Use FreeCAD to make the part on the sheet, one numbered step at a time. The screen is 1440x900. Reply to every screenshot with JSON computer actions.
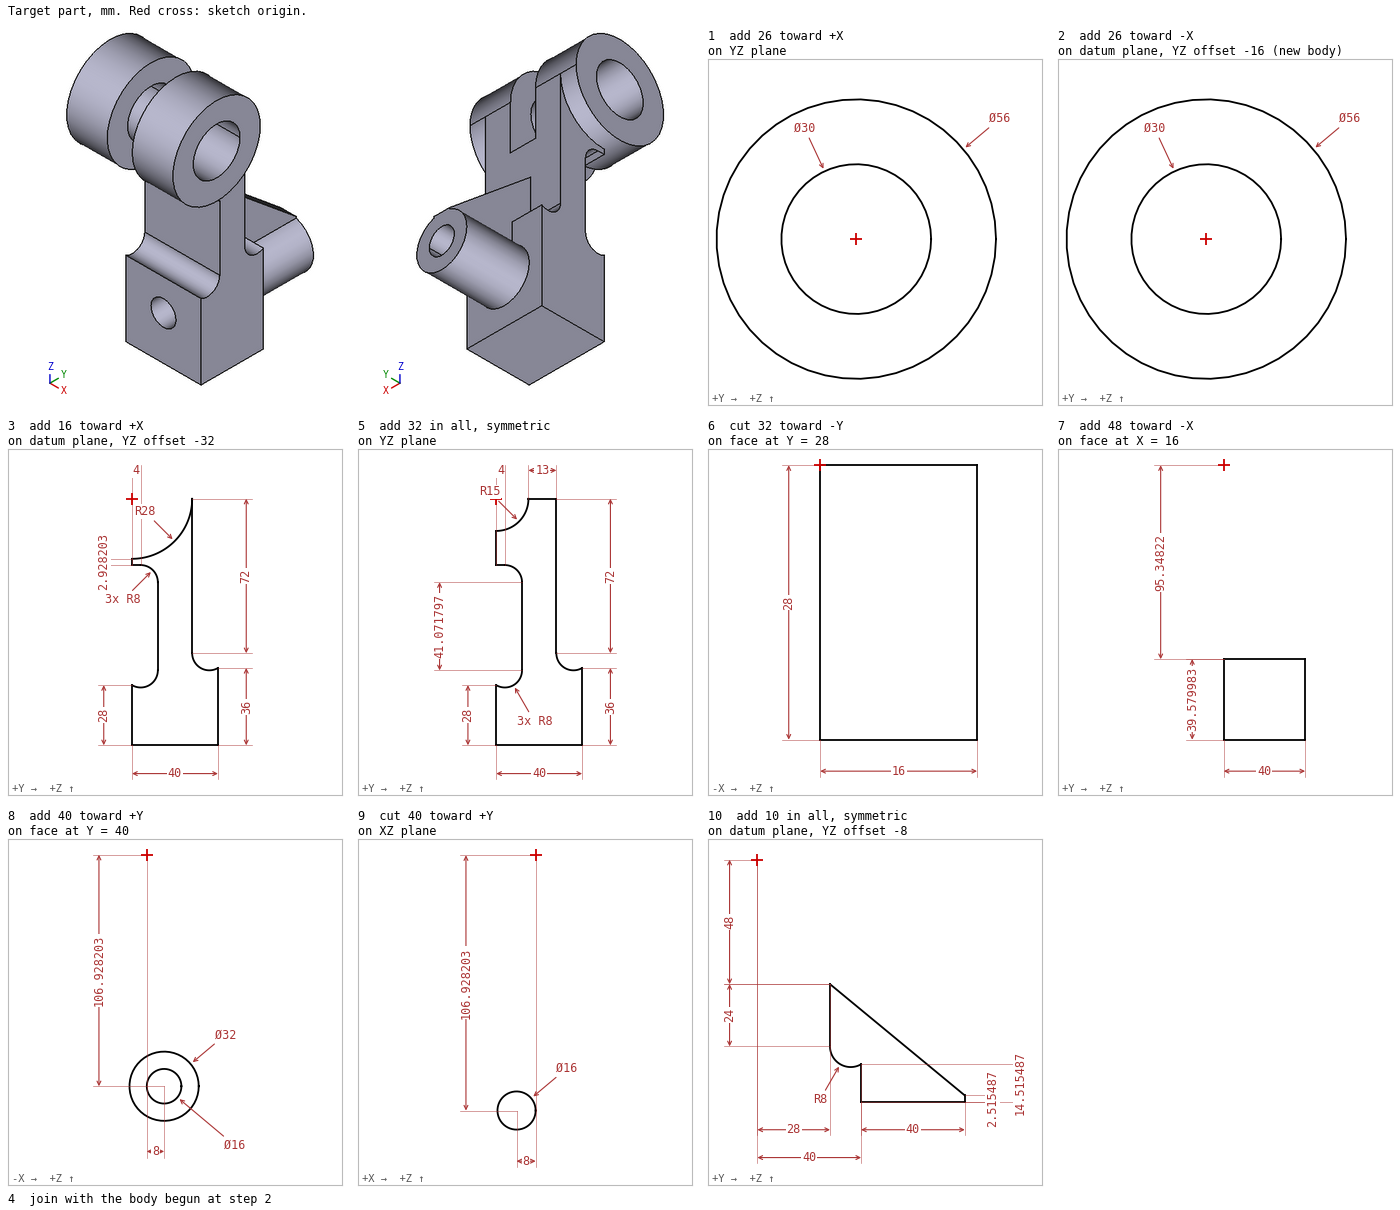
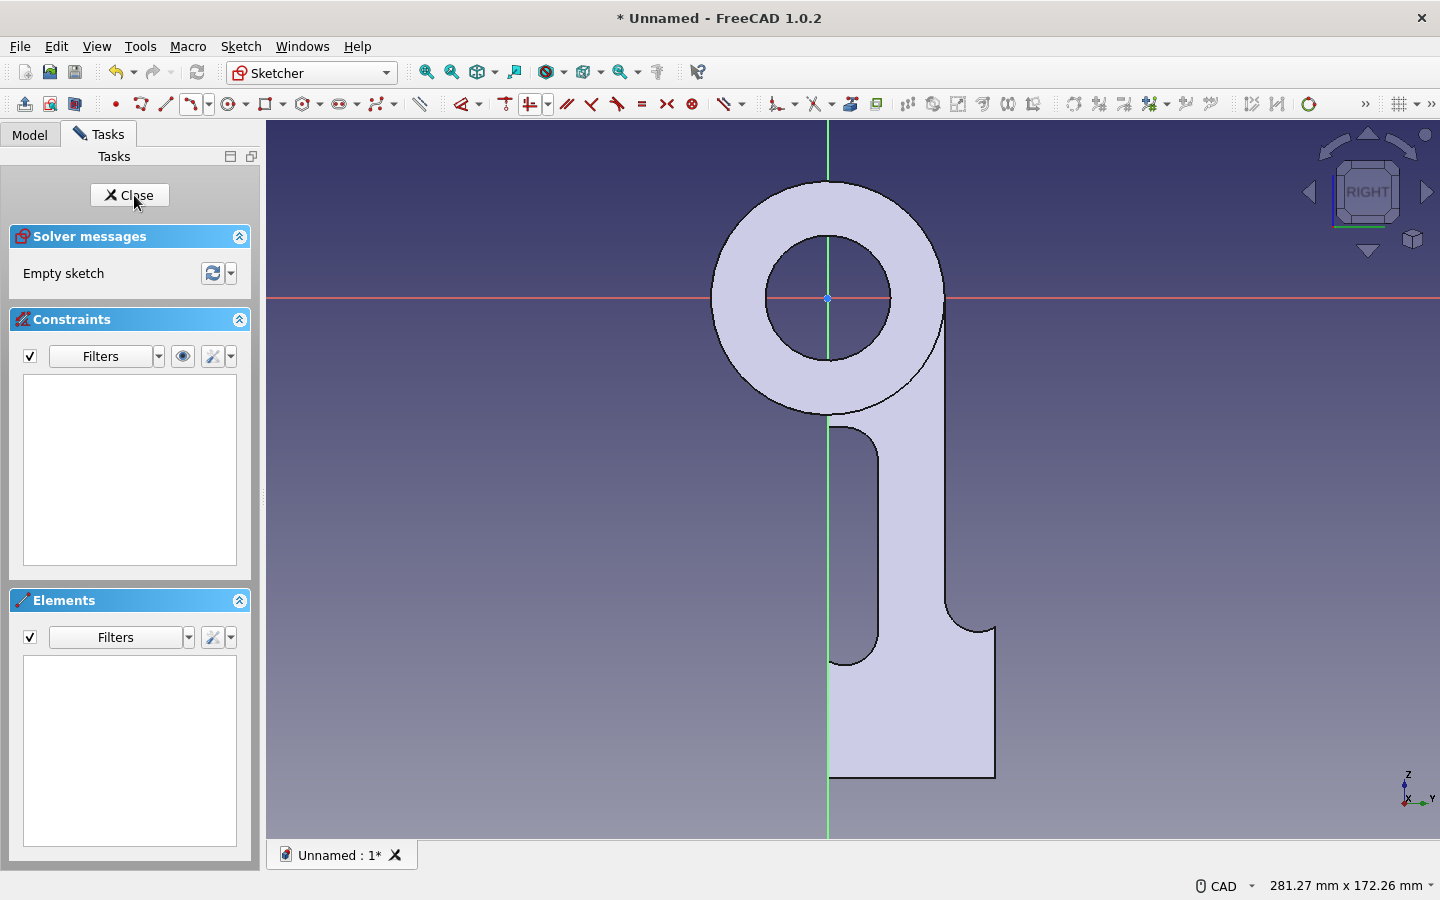
{"action": "left_click", "coordinate": [75, 104]}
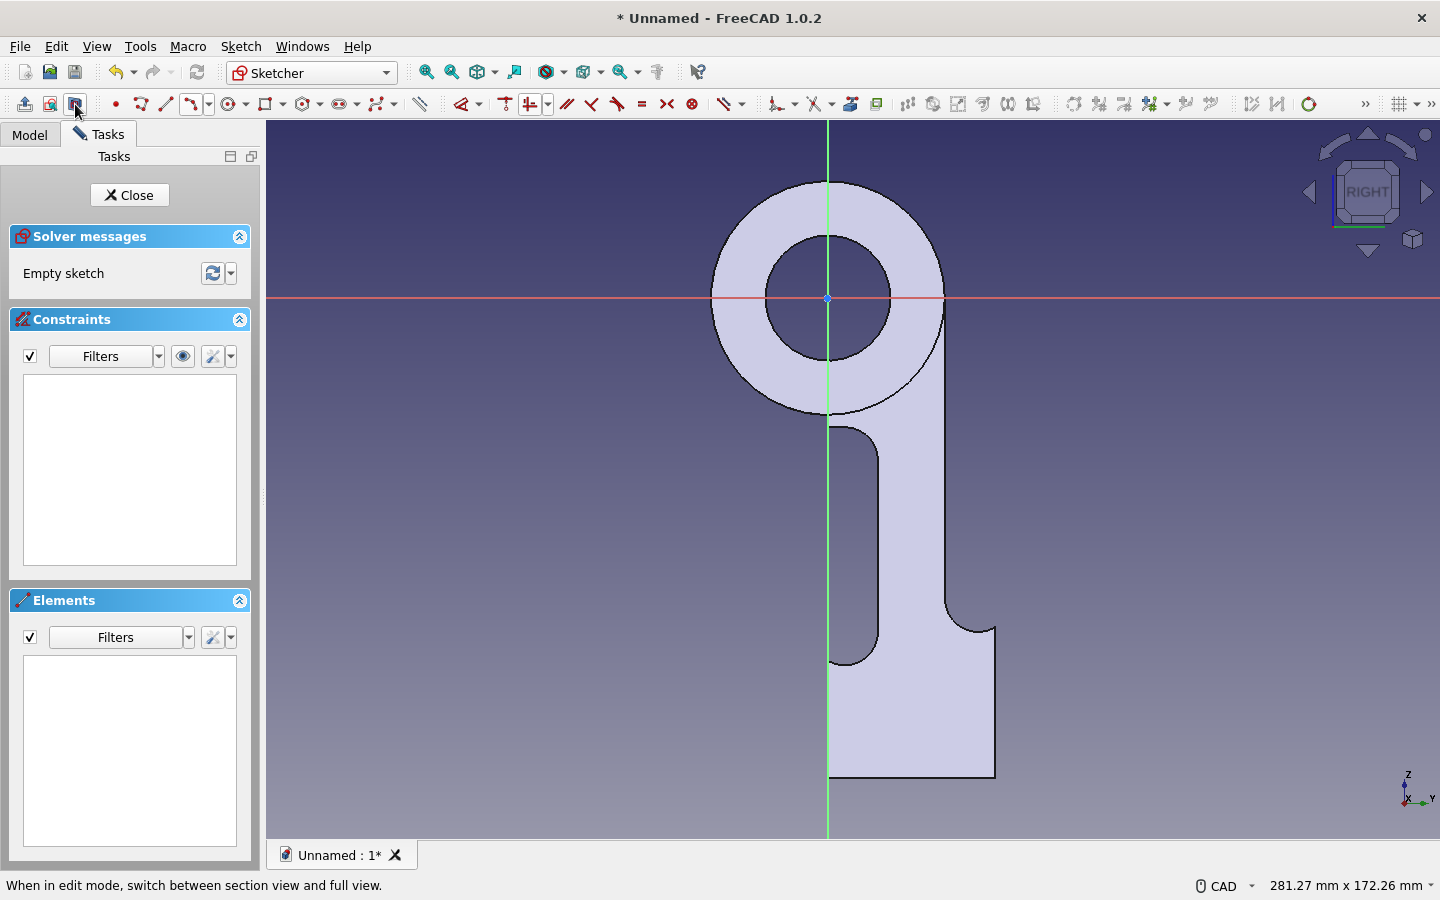
{"action": "key", "text": "g m"}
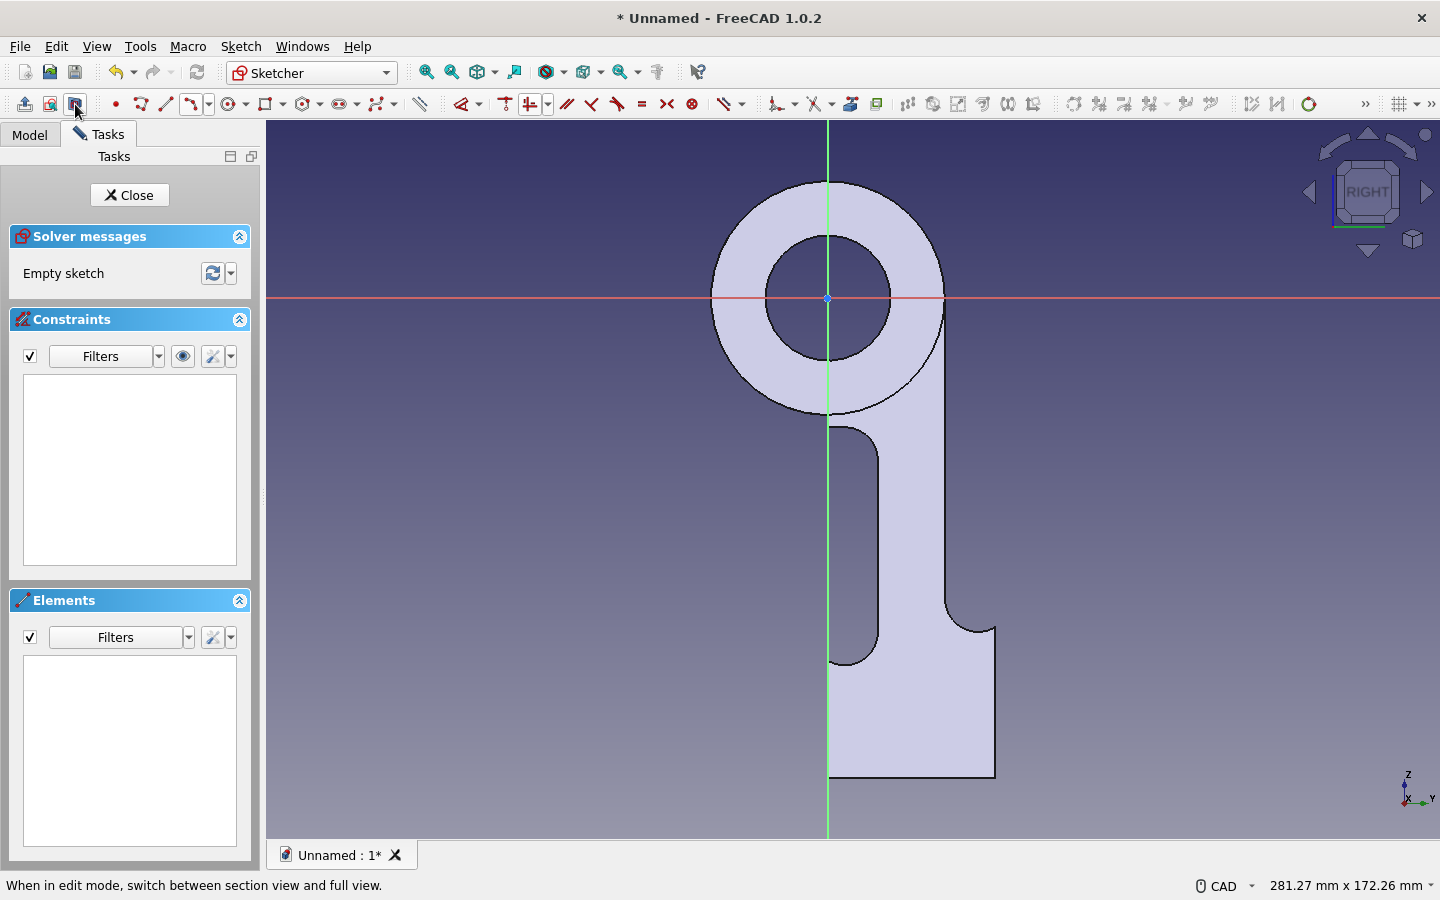
{"action": "left_click", "coordinate": [995, 628]}
{"action": "left_click", "coordinate": [995, 778]}
{"action": "left_click", "coordinate": [828, 778]}
{"action": "left_click", "coordinate": [837, 661]}
{"action": "right_click", "coordinate": [837, 661]}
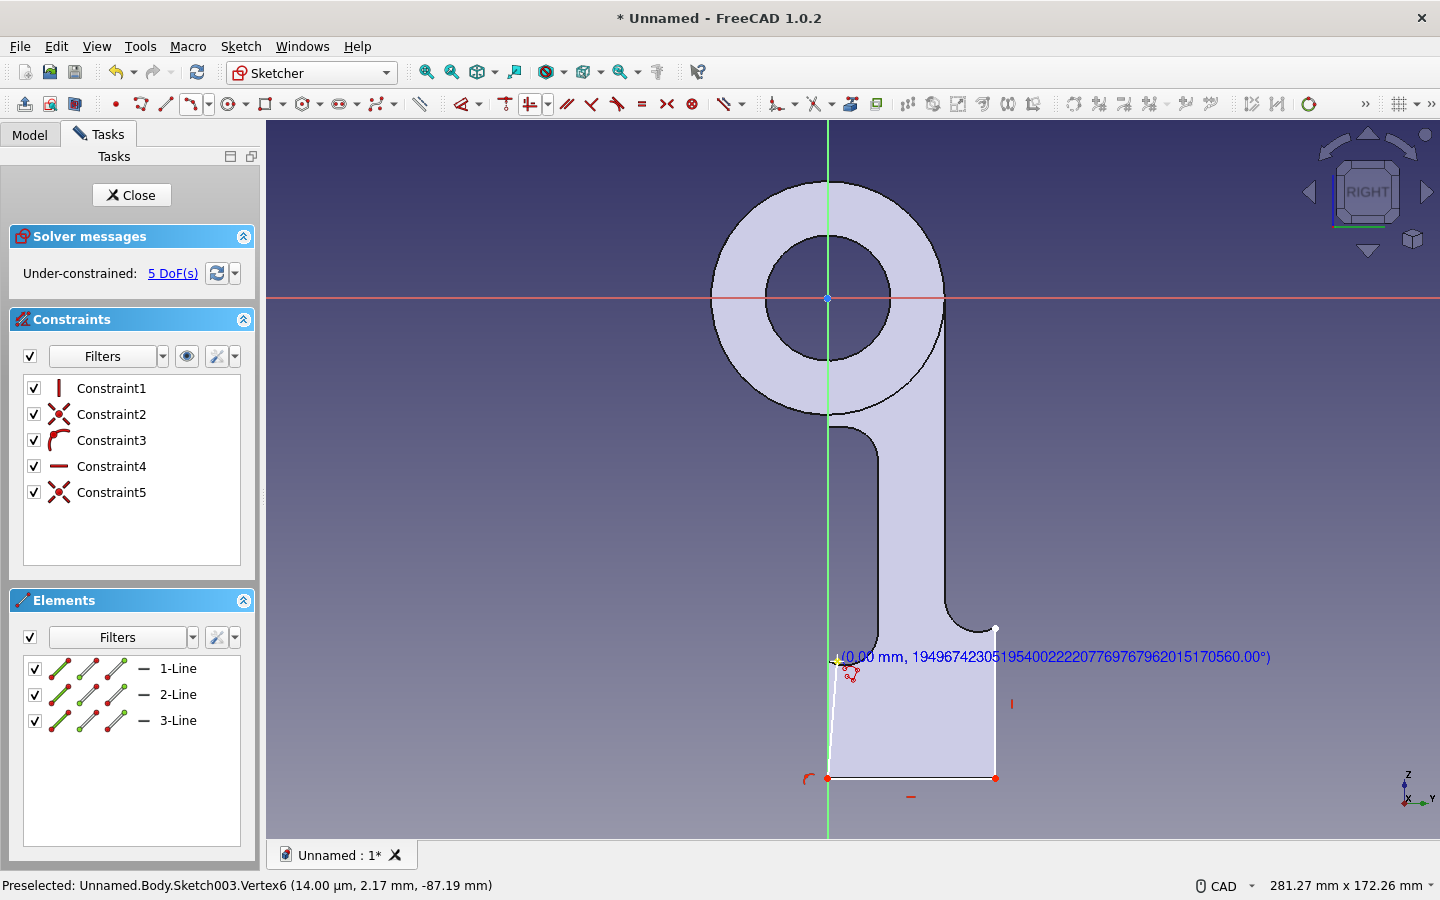
{"action": "left_click", "coordinate": [166, 104]}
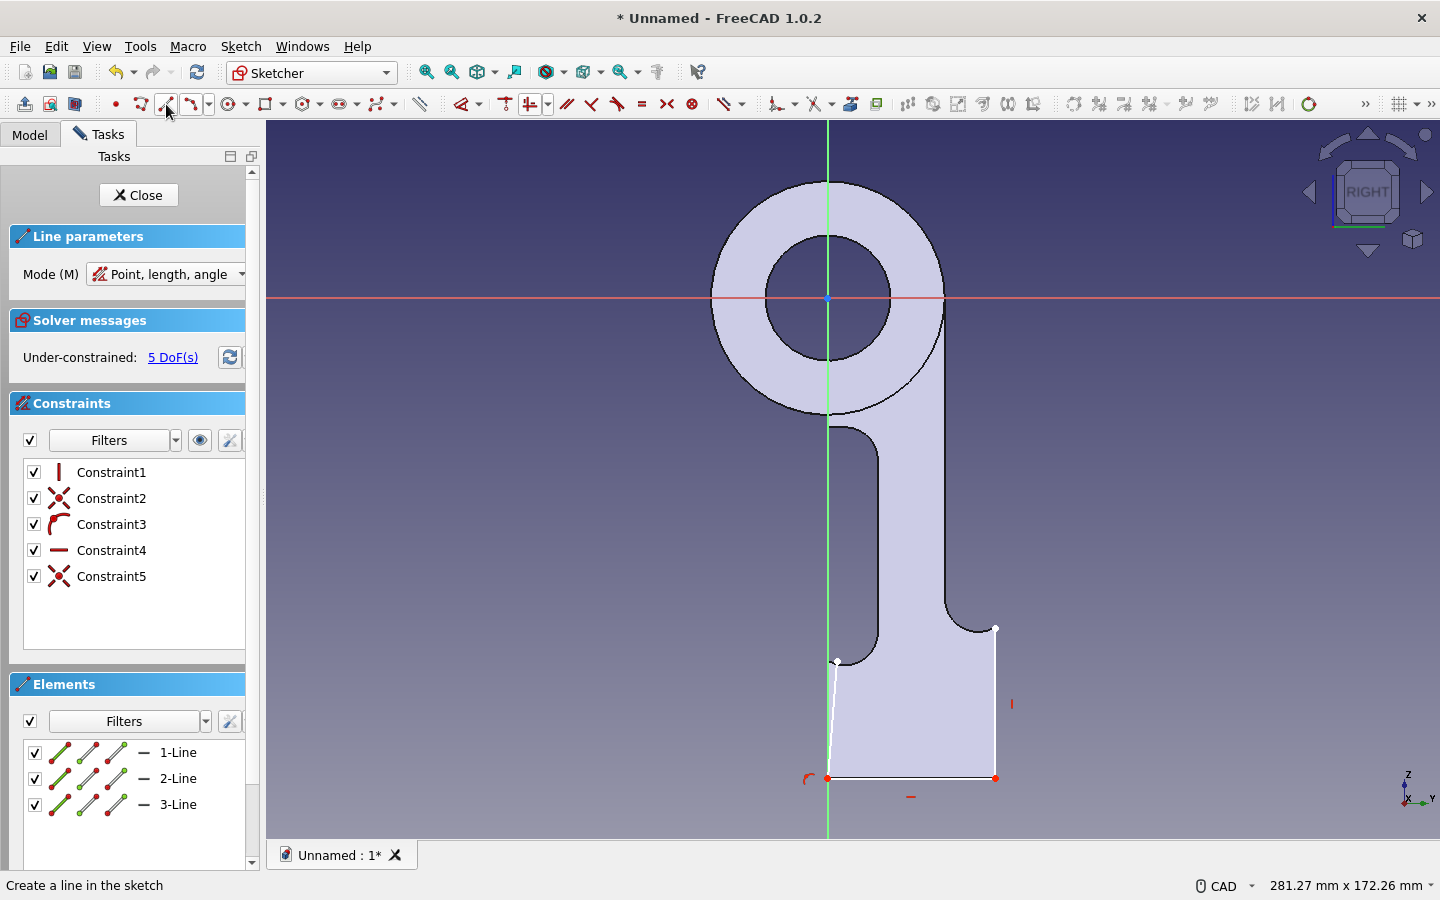
{"action": "left_click", "coordinate": [878, 632]}
{"action": "left_click", "coordinate": [878, 461]}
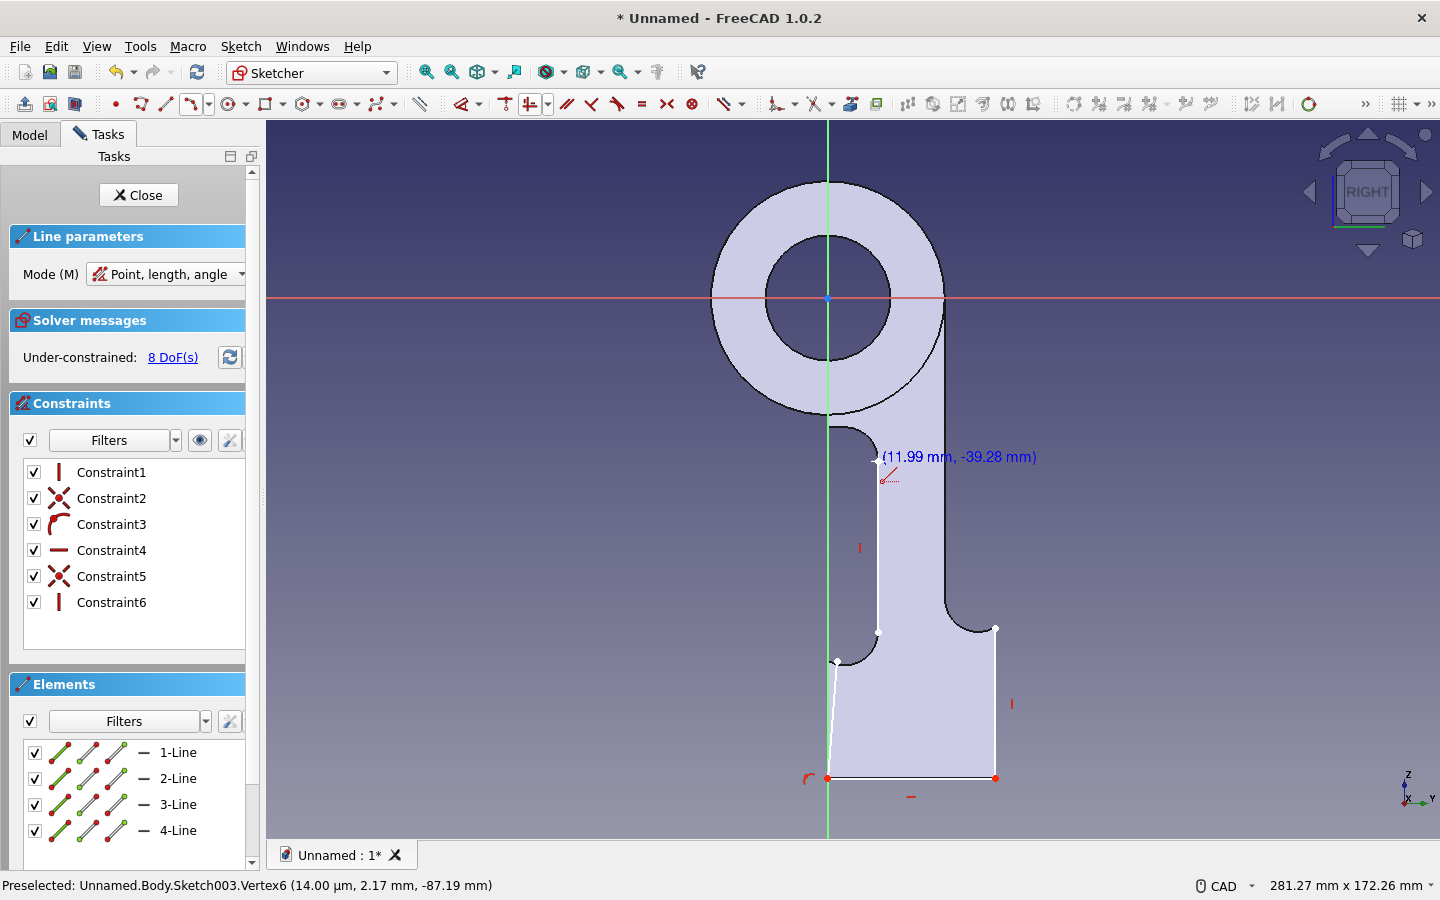
{"action": "key", "text": "g m"}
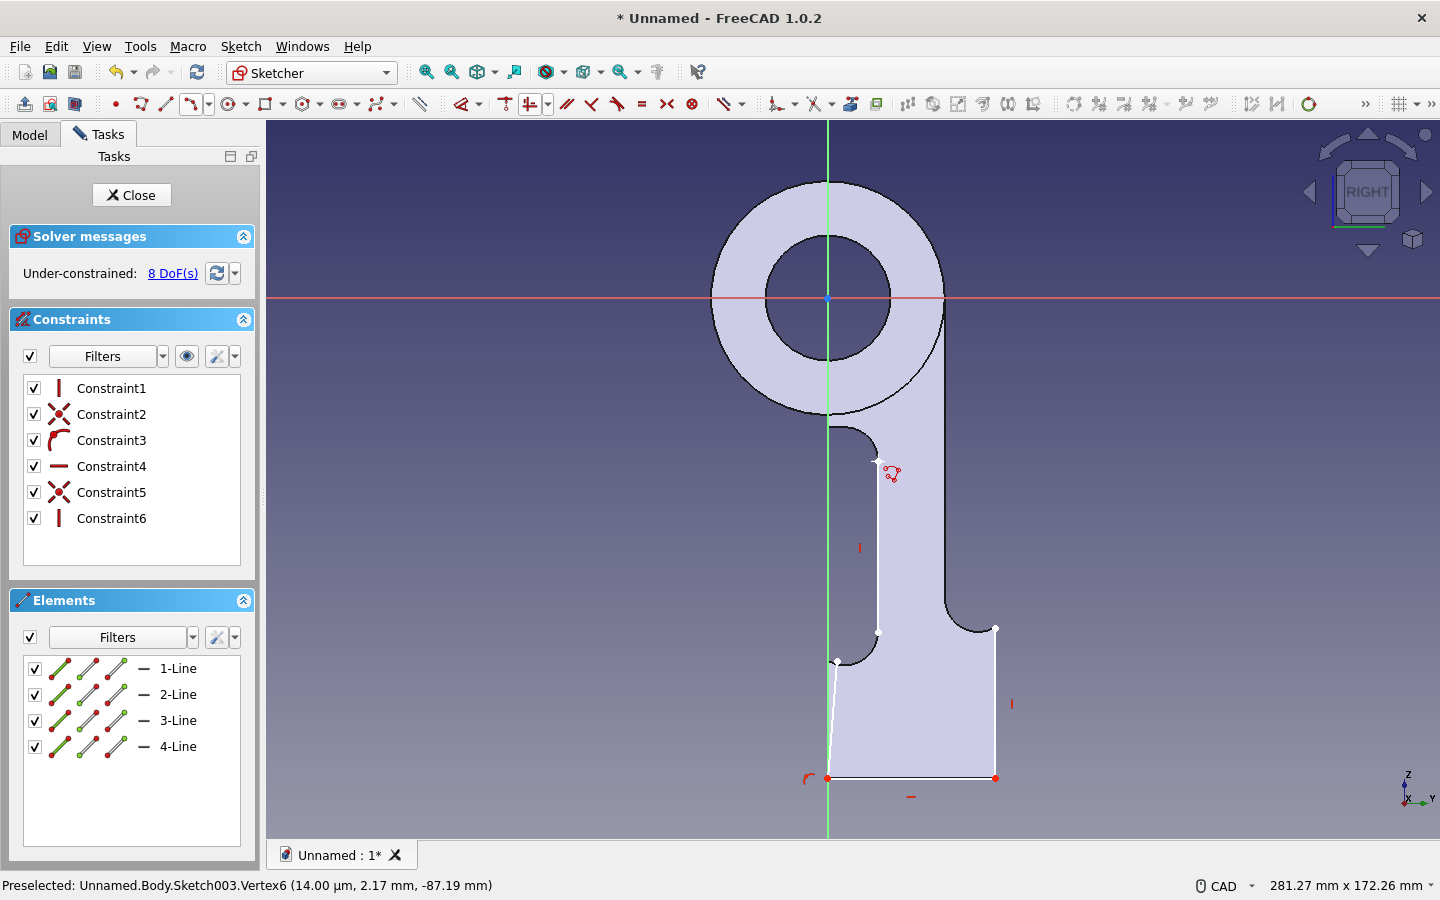
{"action": "left_click", "coordinate": [845, 427]}
{"action": "left_click", "coordinate": [828, 427]}
{"action": "left_click", "coordinate": [837, 361]}
{"action": "right_click", "coordinate": [837, 361]}